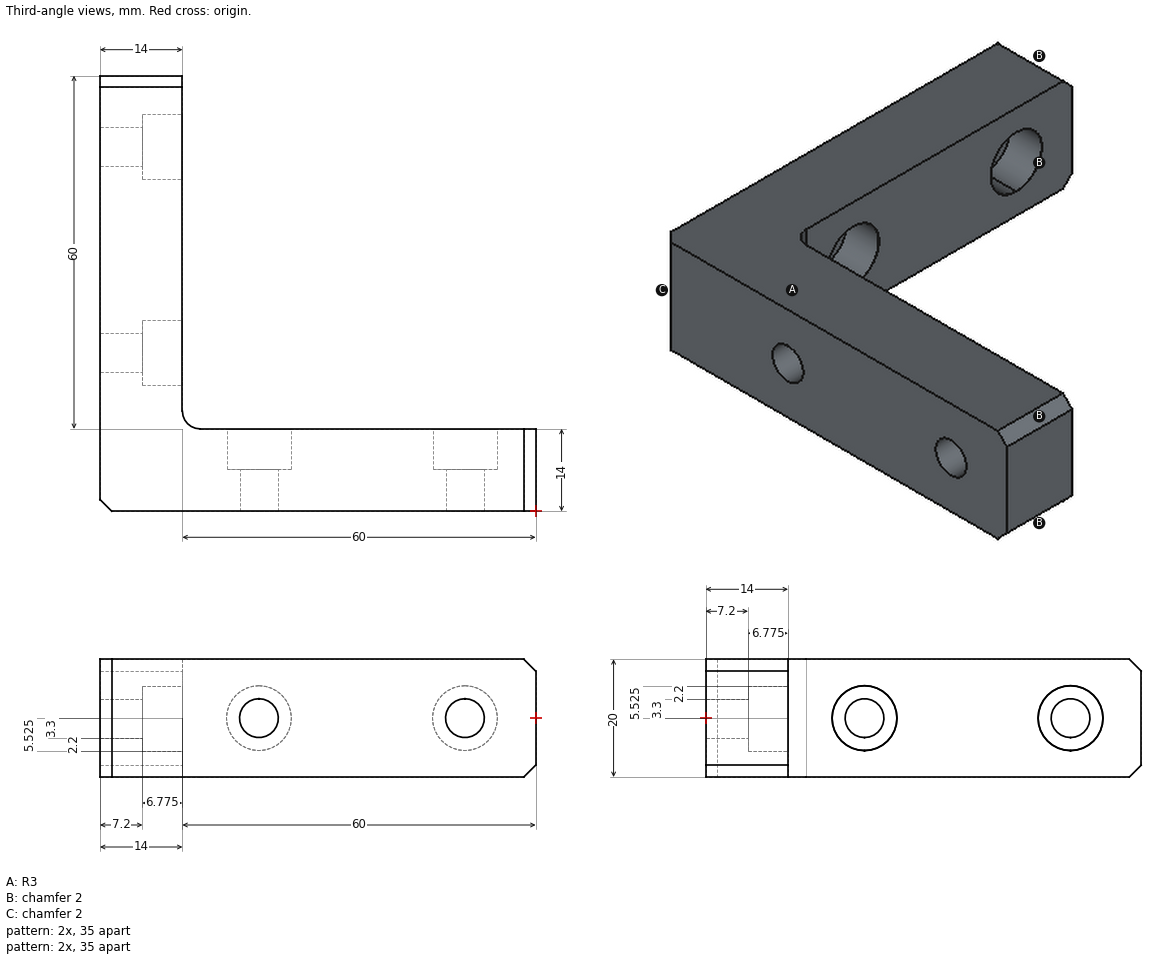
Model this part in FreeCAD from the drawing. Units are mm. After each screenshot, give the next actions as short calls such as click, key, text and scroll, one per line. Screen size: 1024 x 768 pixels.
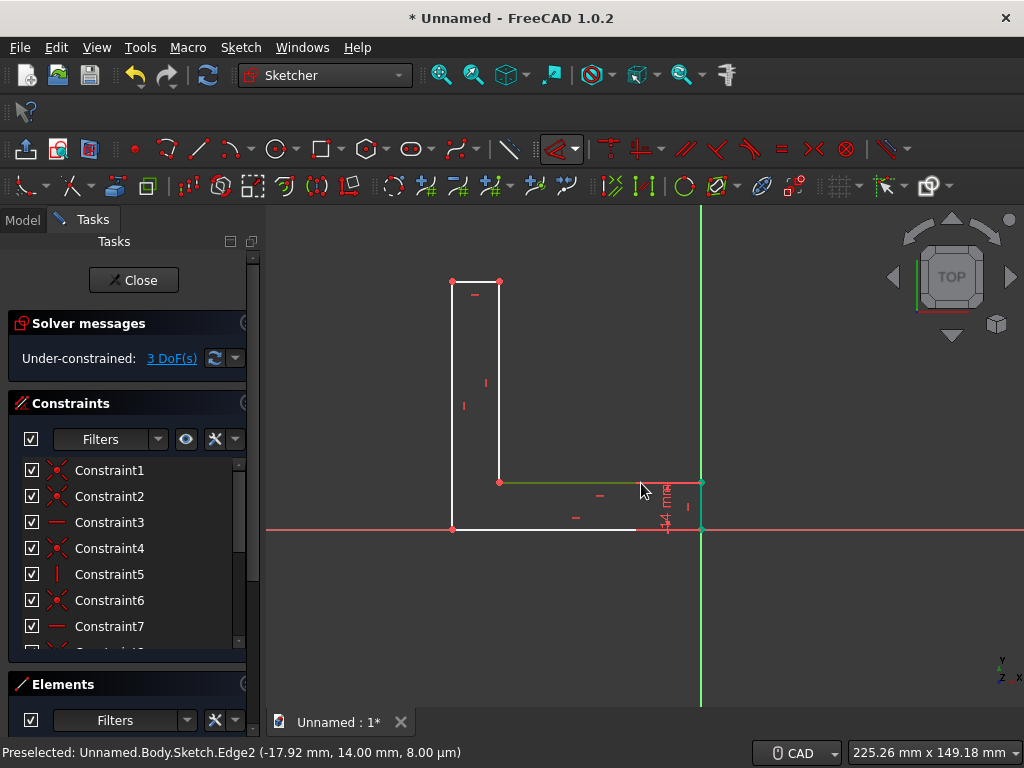
click(578, 150)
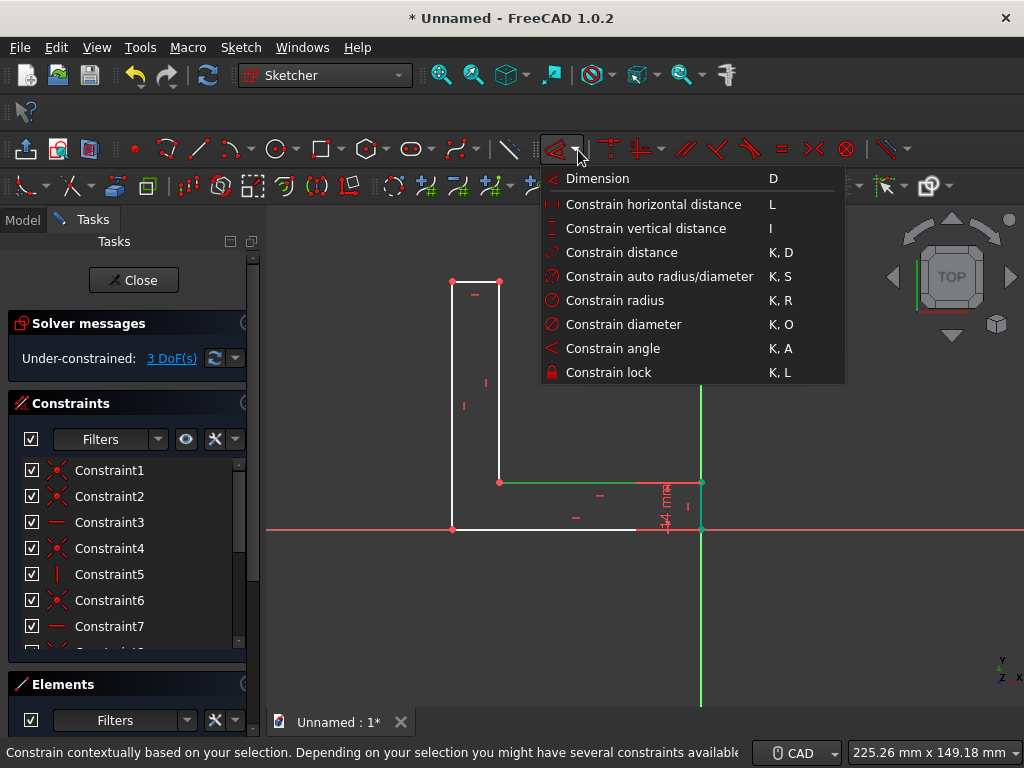
click(693, 204)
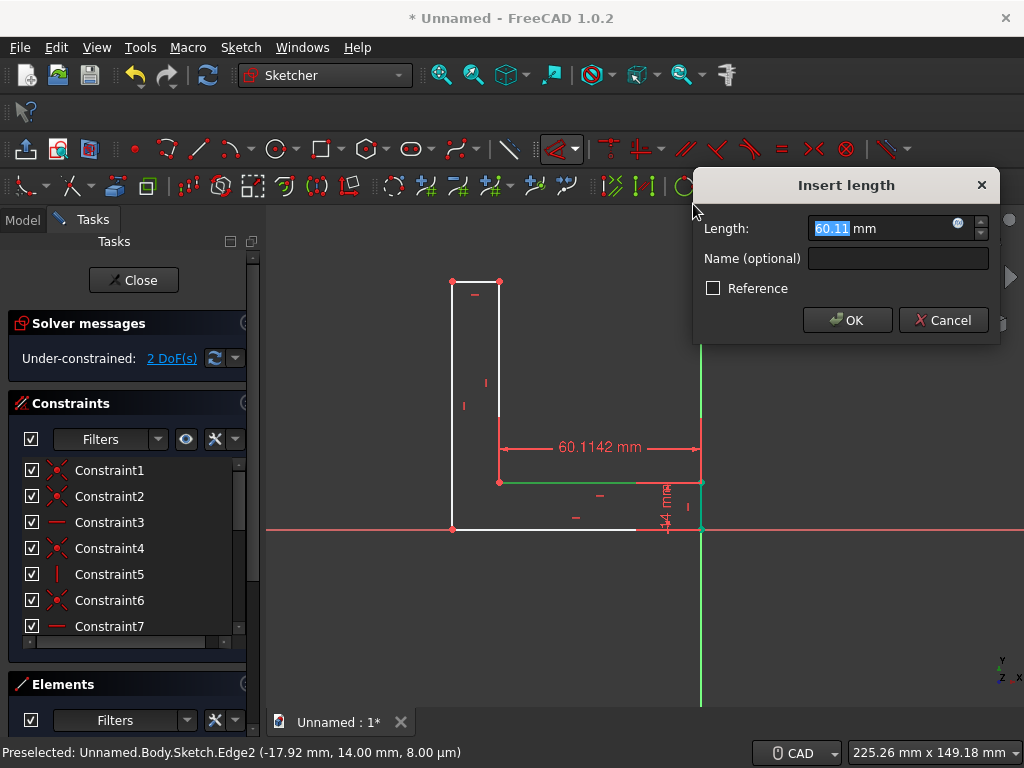
text(60)
key(Return)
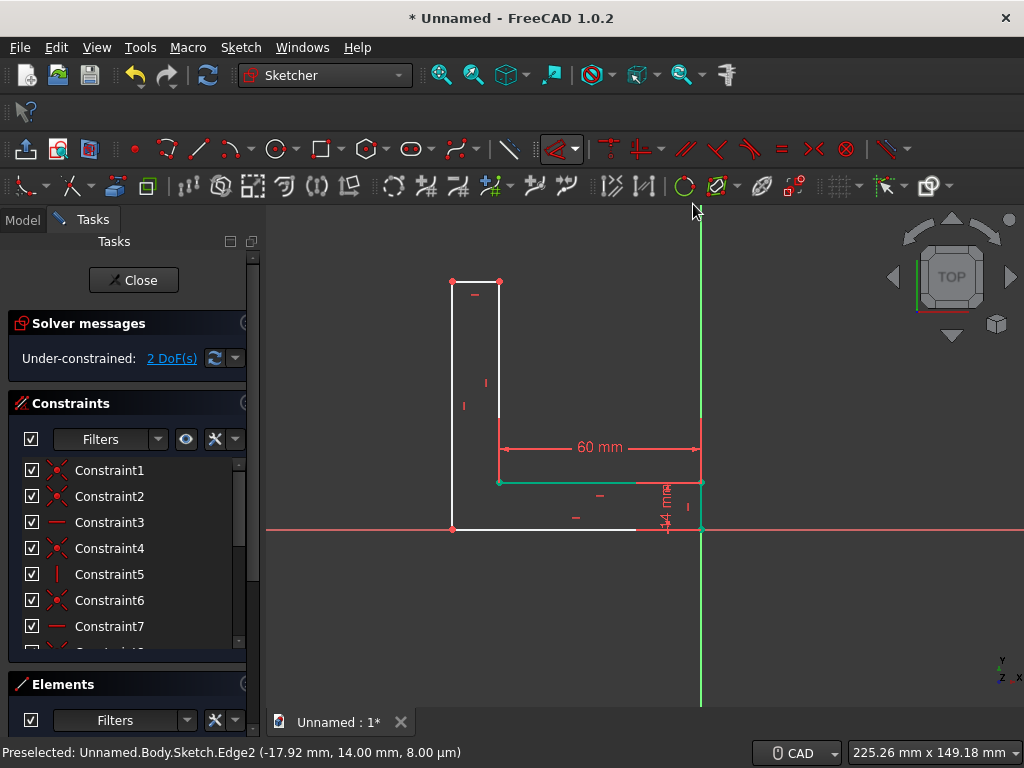
click(499, 423)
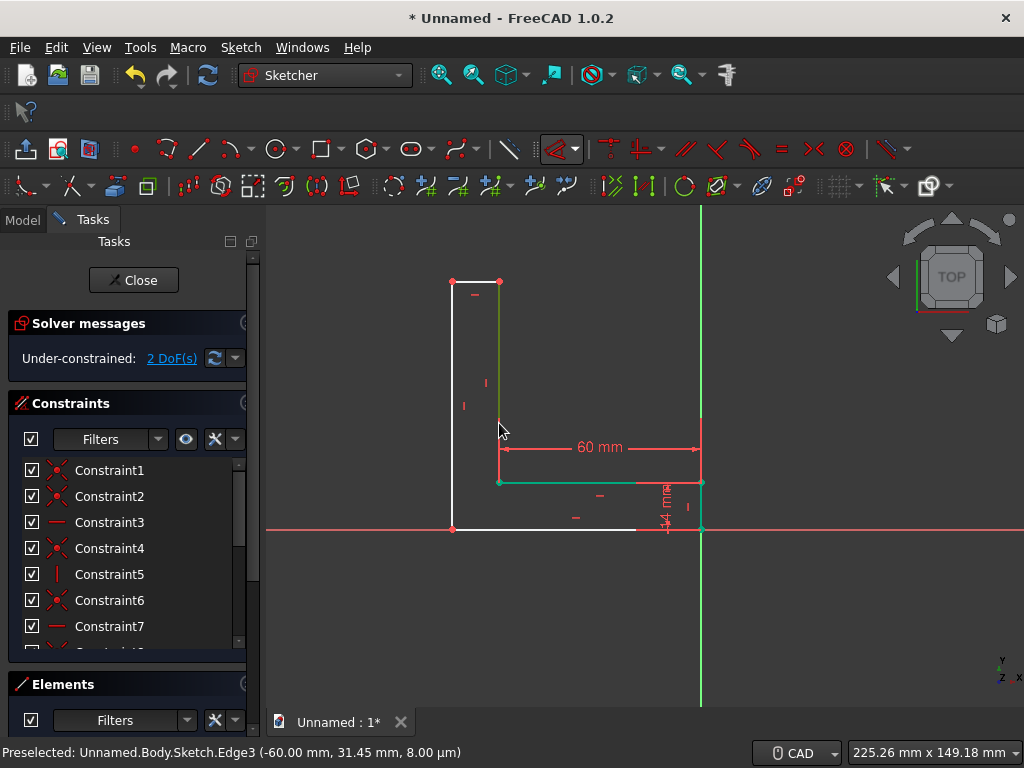
click(578, 150)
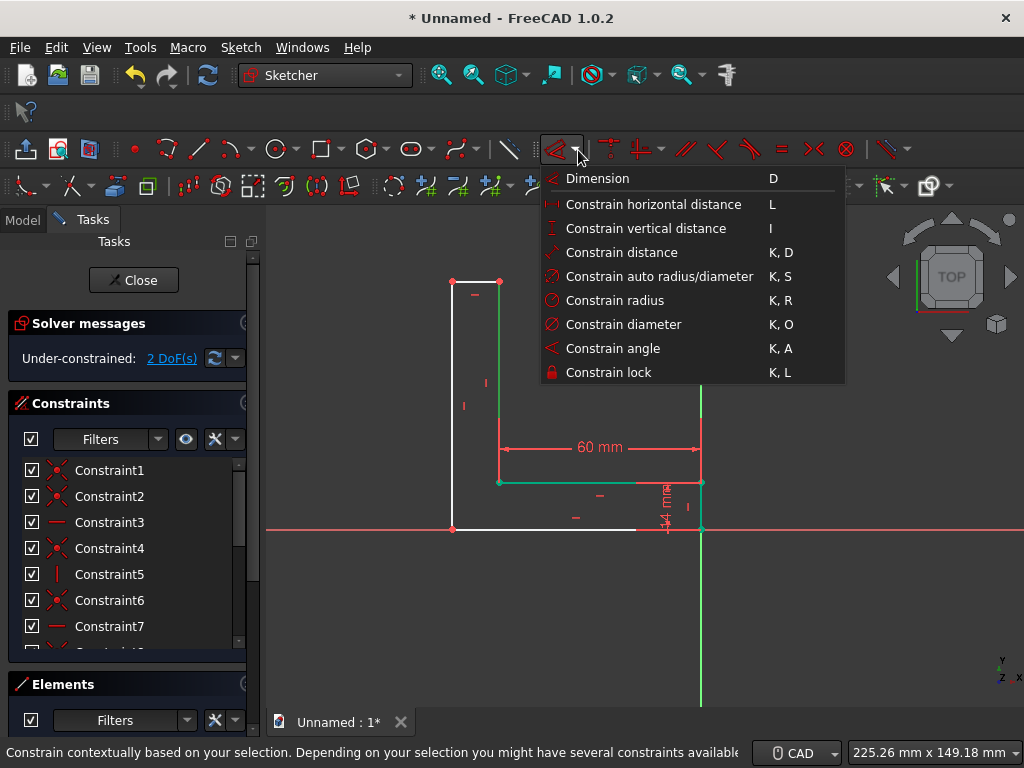
click(693, 228)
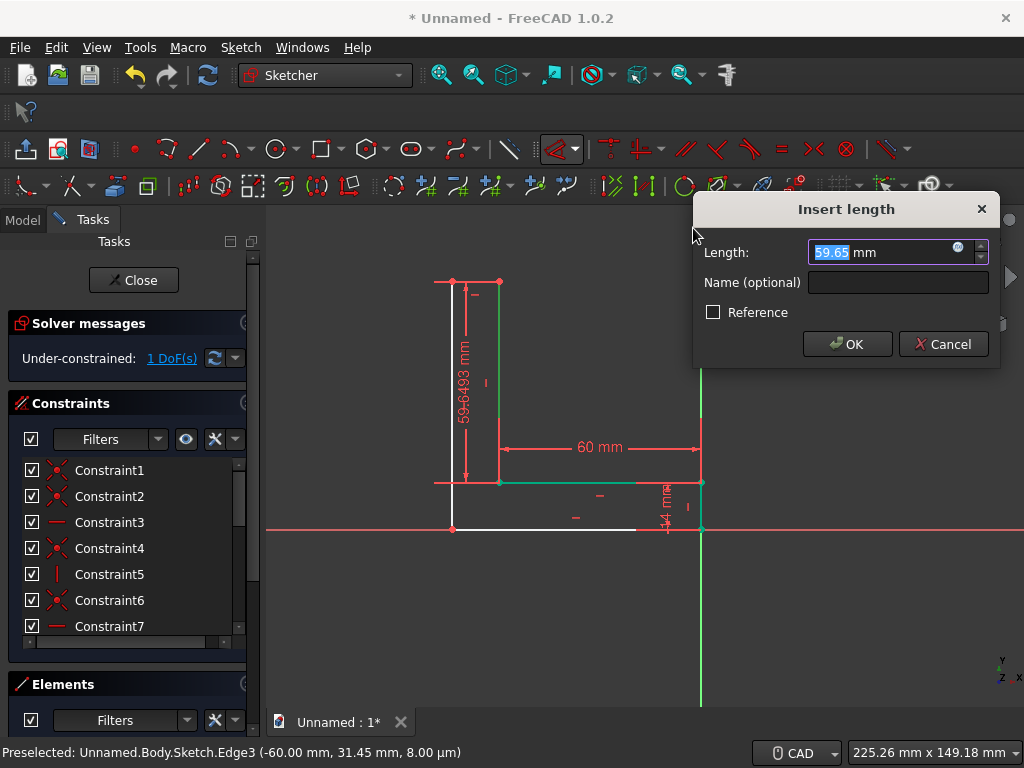
text(60)
key(Return)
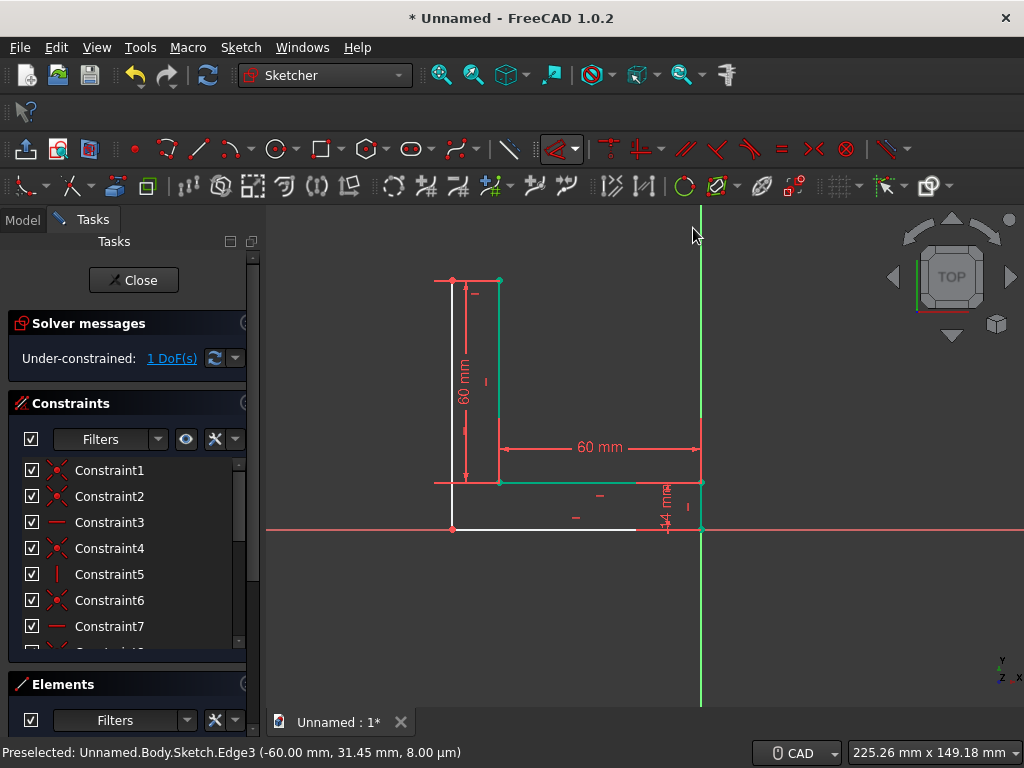
click(485, 281)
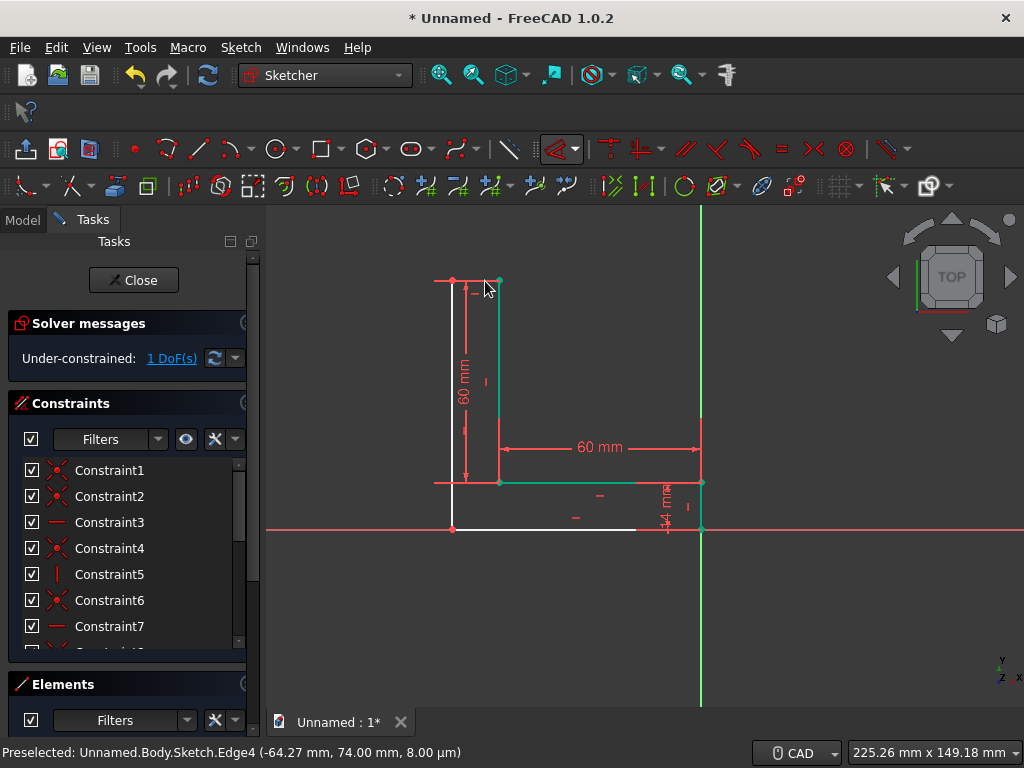
key(l)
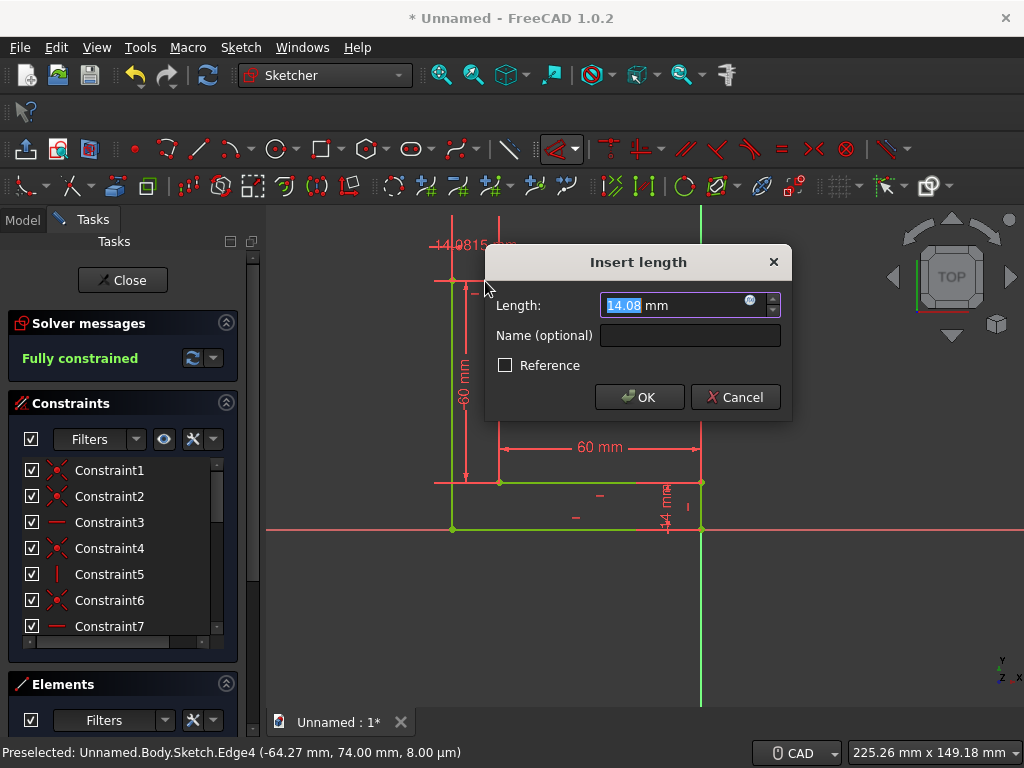
text(14)
key(Return)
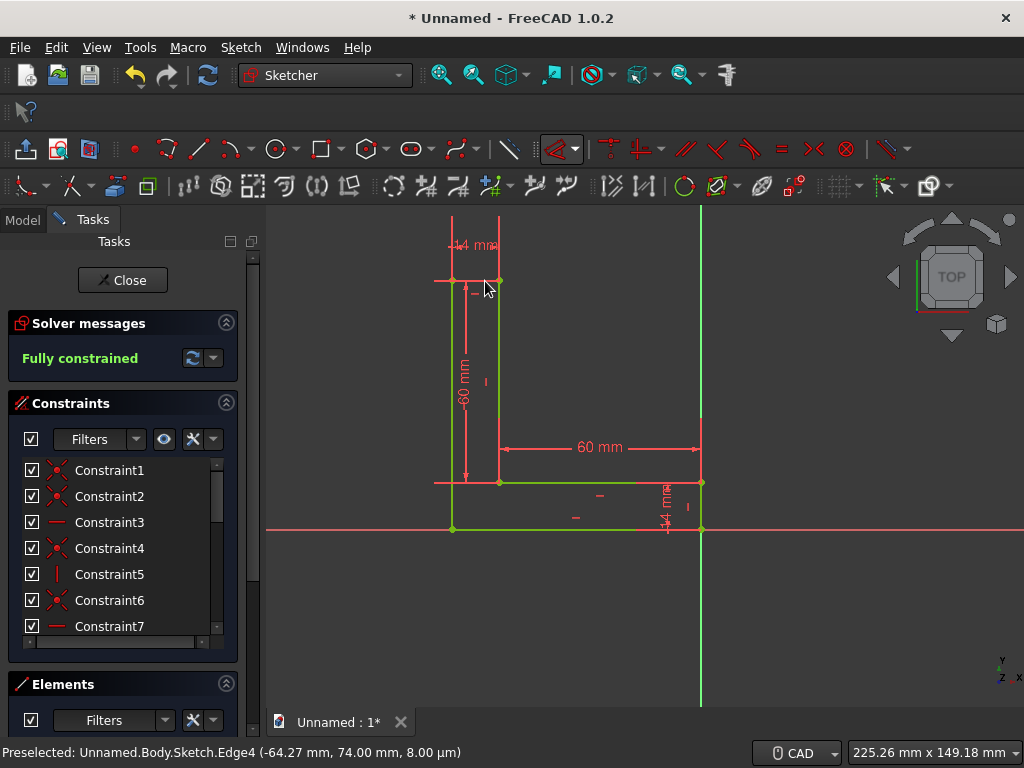
click(123, 280)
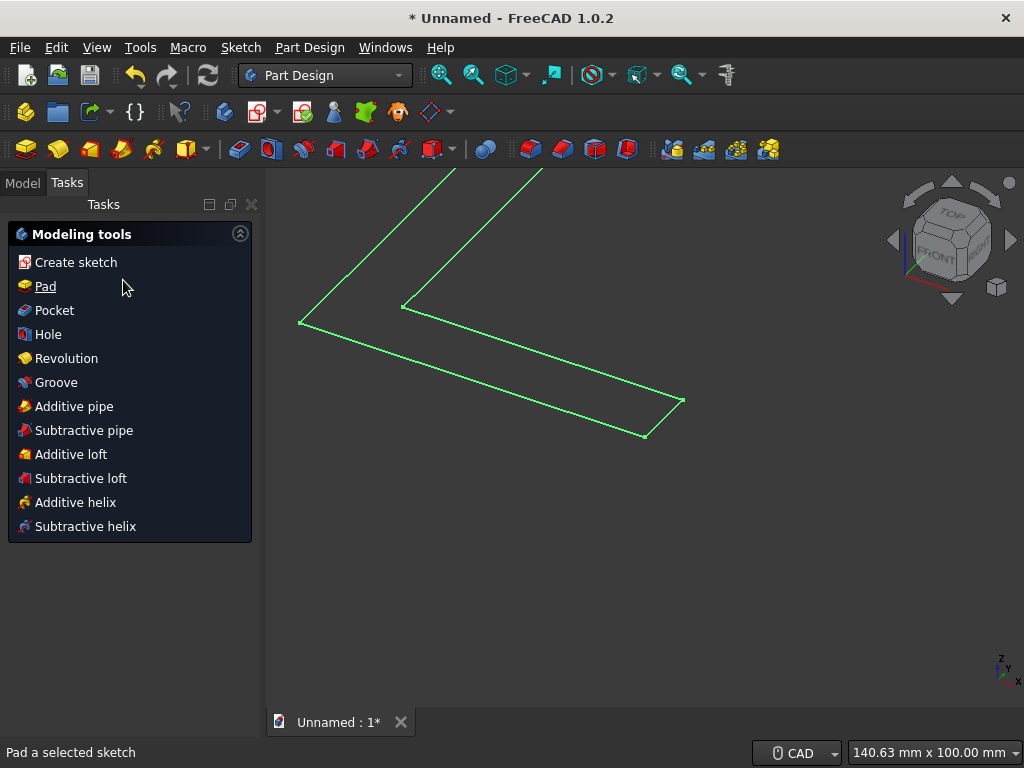
click(26, 150)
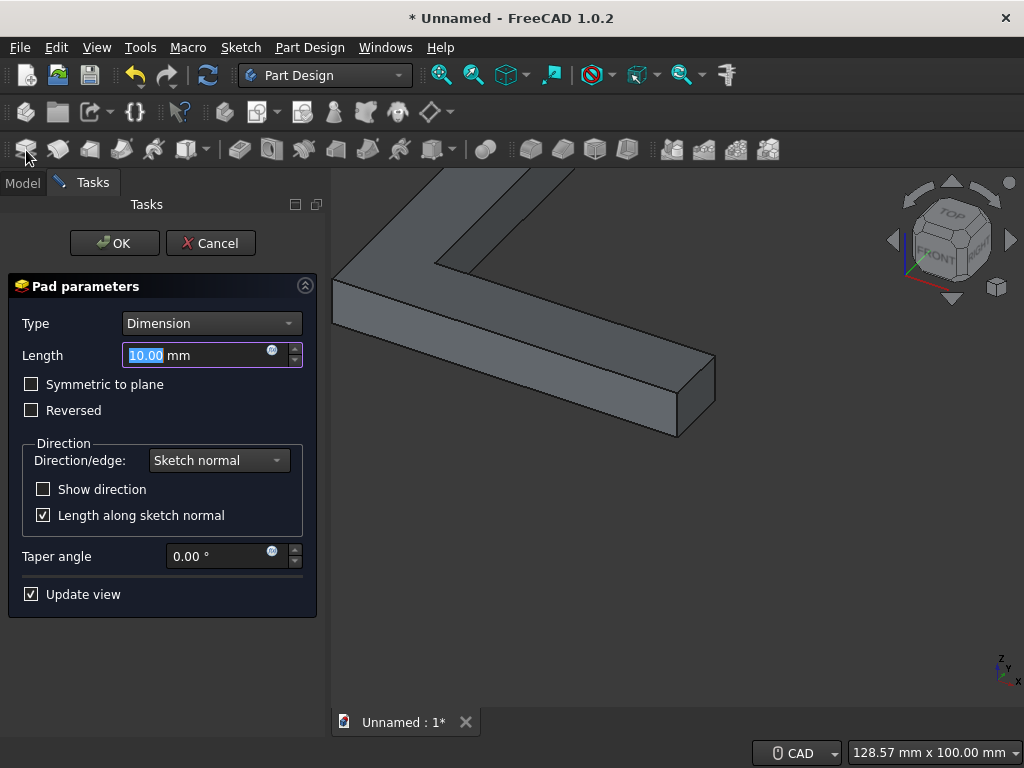
text(20)
key(Tab)